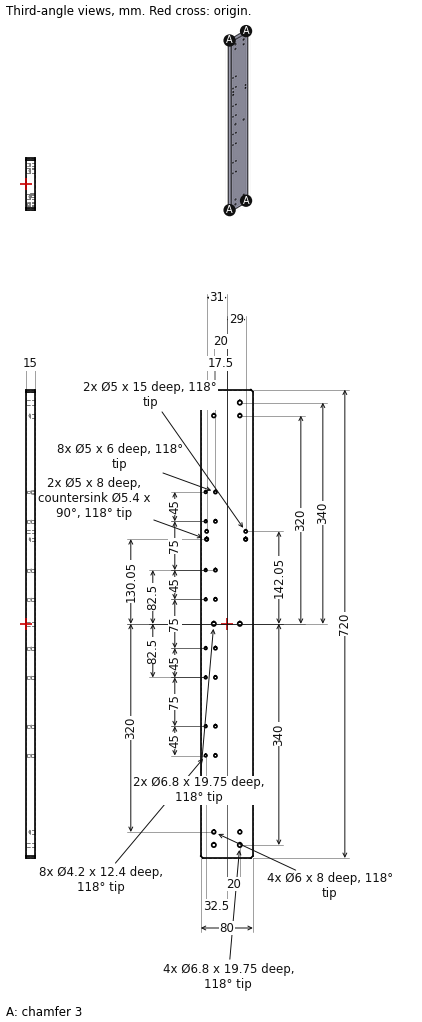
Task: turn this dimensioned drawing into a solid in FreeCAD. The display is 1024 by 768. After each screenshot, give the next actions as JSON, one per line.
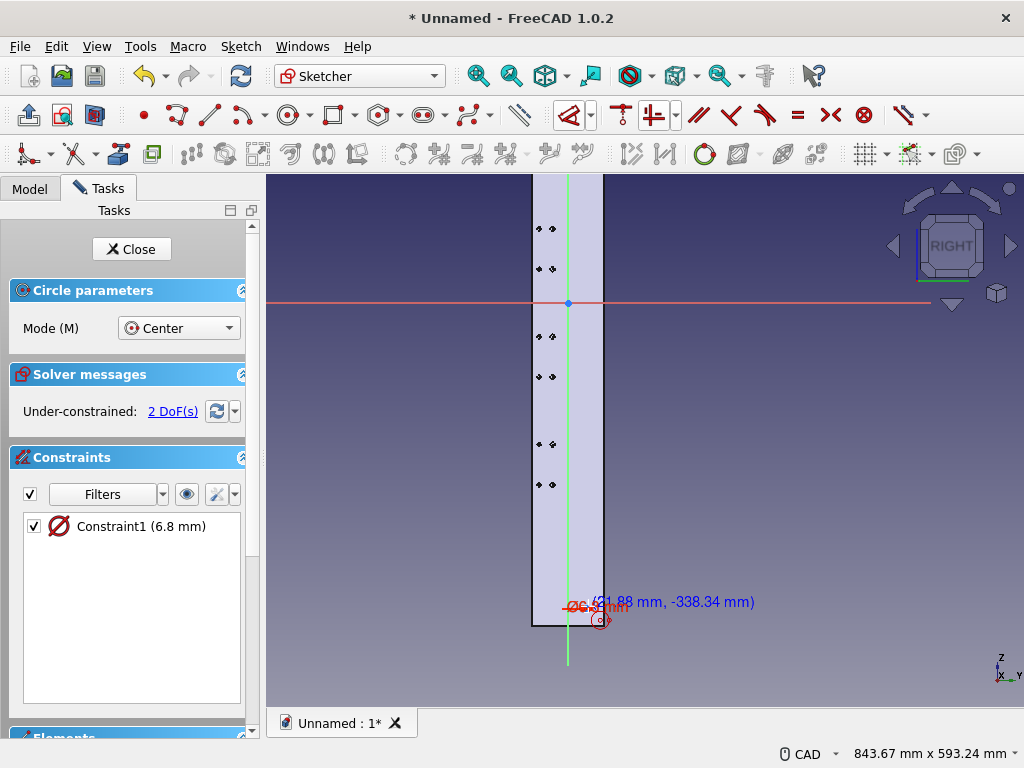
{"action": "scroll", "coordinate": [586, 608], "scroll_direction": "down", "scroll_amount": 3}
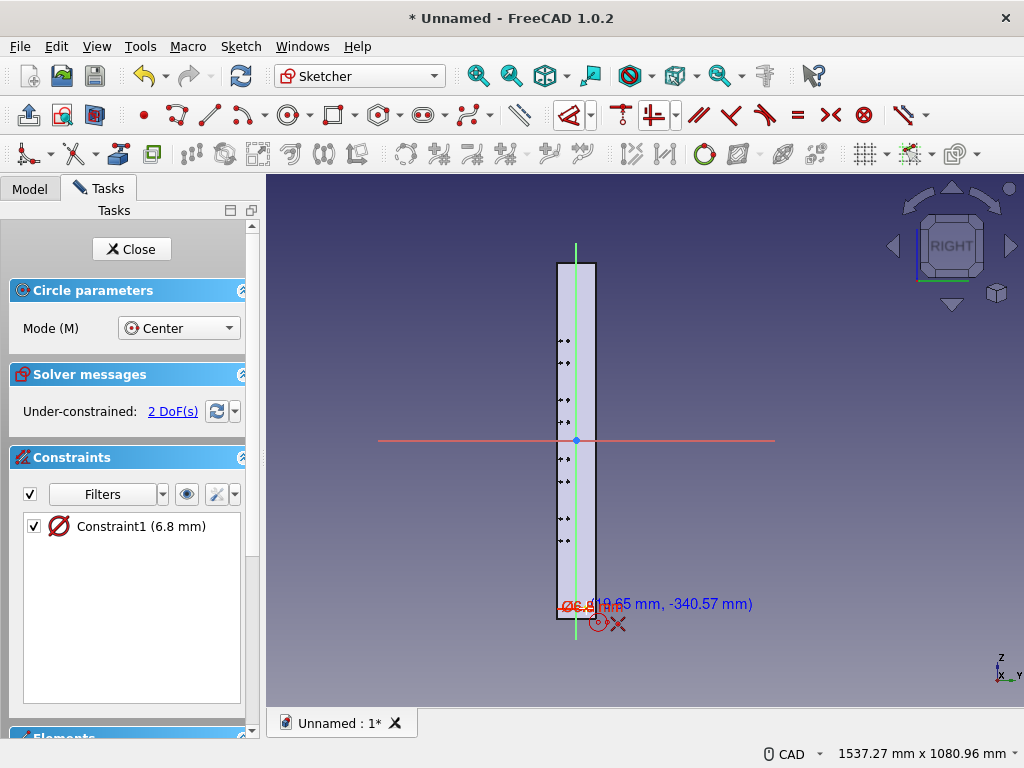
{"action": "scroll", "coordinate": [586, 273], "scroll_direction": "up", "scroll_amount": 14}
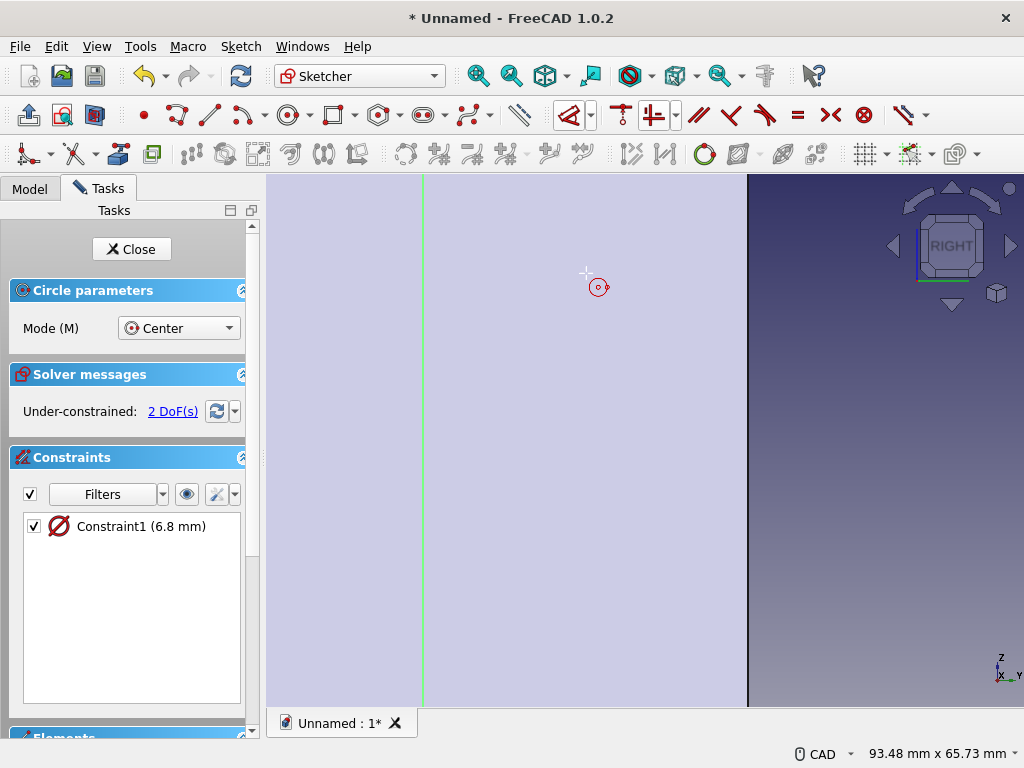
{"action": "scroll", "coordinate": [586, 273], "scroll_direction": "down", "scroll_amount": 14}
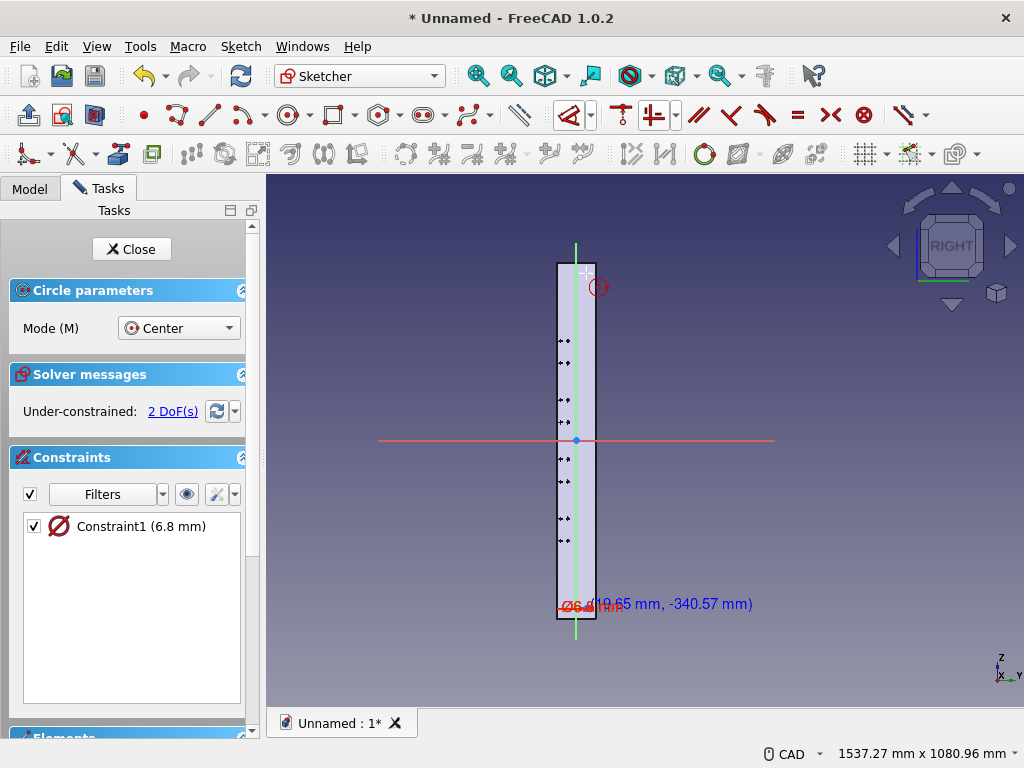
{"action": "scroll", "coordinate": [586, 273], "scroll_direction": "up", "scroll_amount": 3}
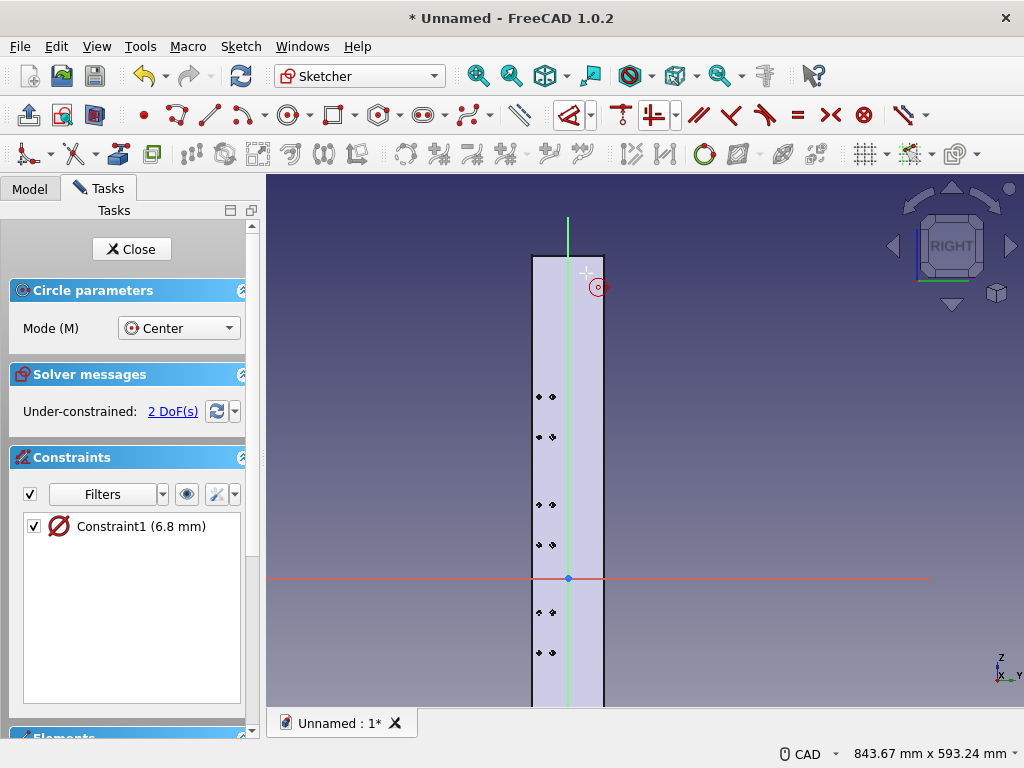
{"action": "left_click", "coordinate": [586, 273]}
{"action": "mouse_move", "coordinate": [588, 271]}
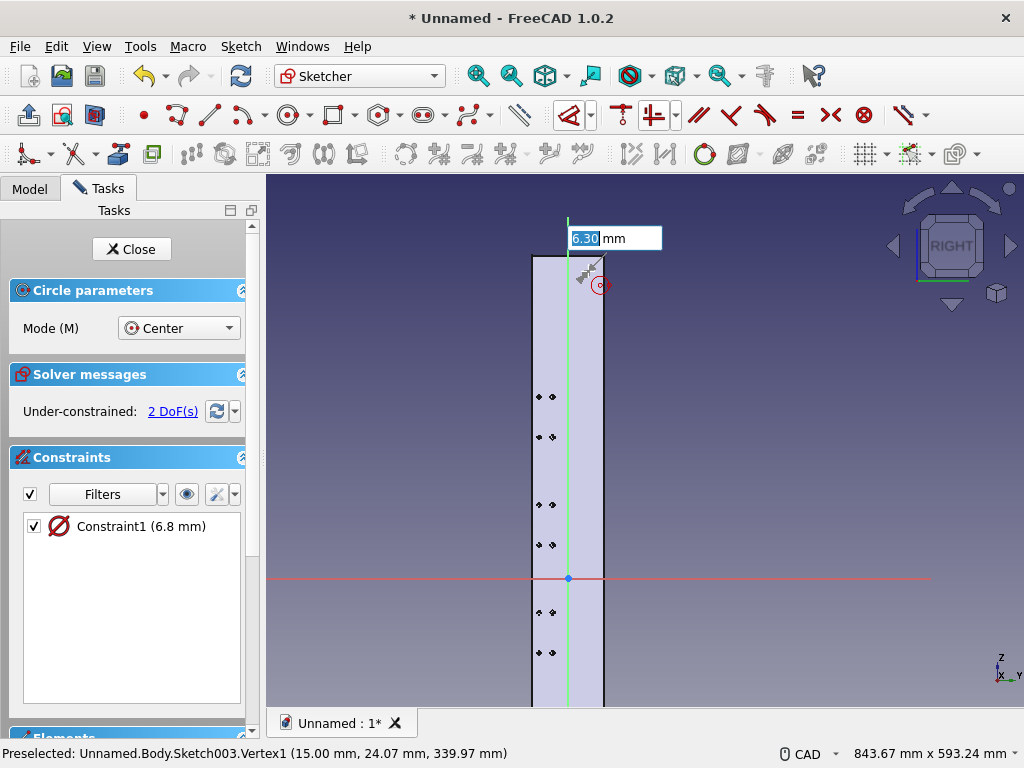
{"action": "type", "text": "6.8"}
{"action": "key", "text": "Return"}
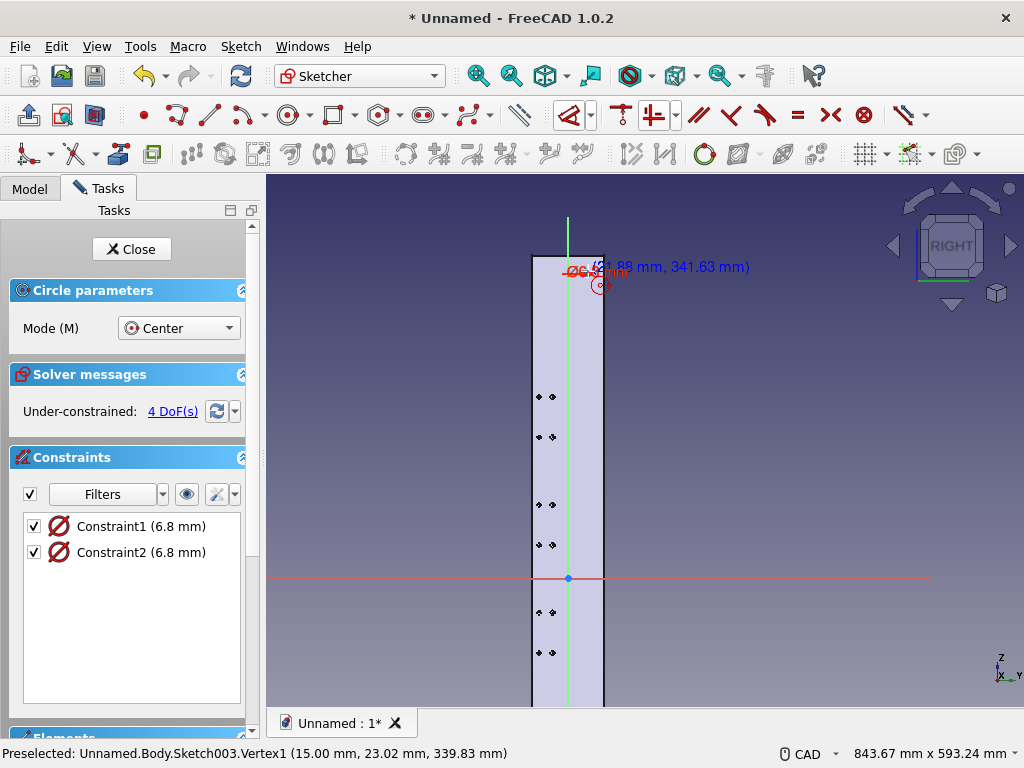
{"action": "scroll", "coordinate": [550, 273], "scroll_direction": "up", "scroll_amount": 11}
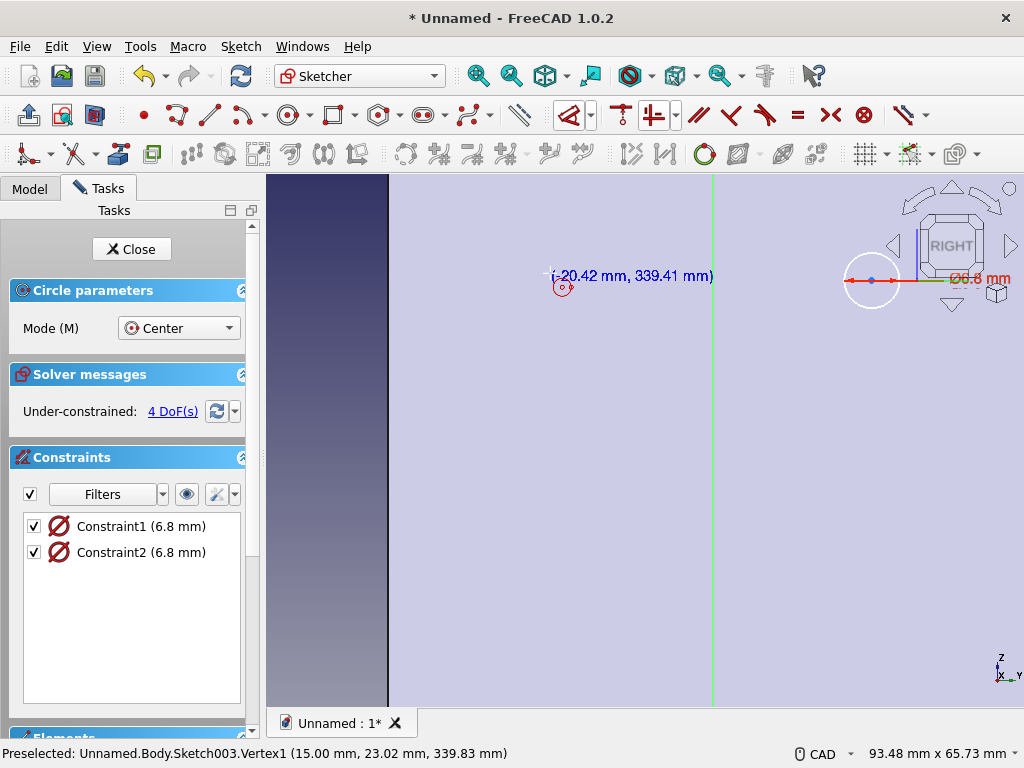
{"action": "scroll", "coordinate": [568, 273], "scroll_direction": "down", "scroll_amount": 14}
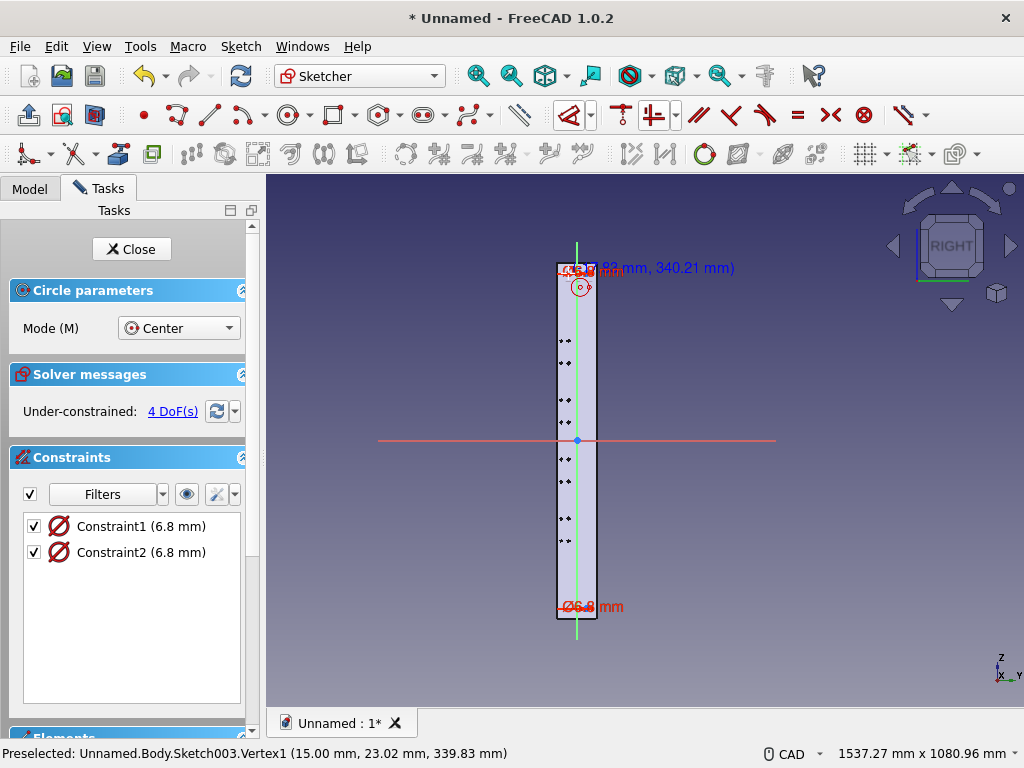
{"action": "scroll", "coordinate": [567, 273], "scroll_direction": "up", "scroll_amount": 3}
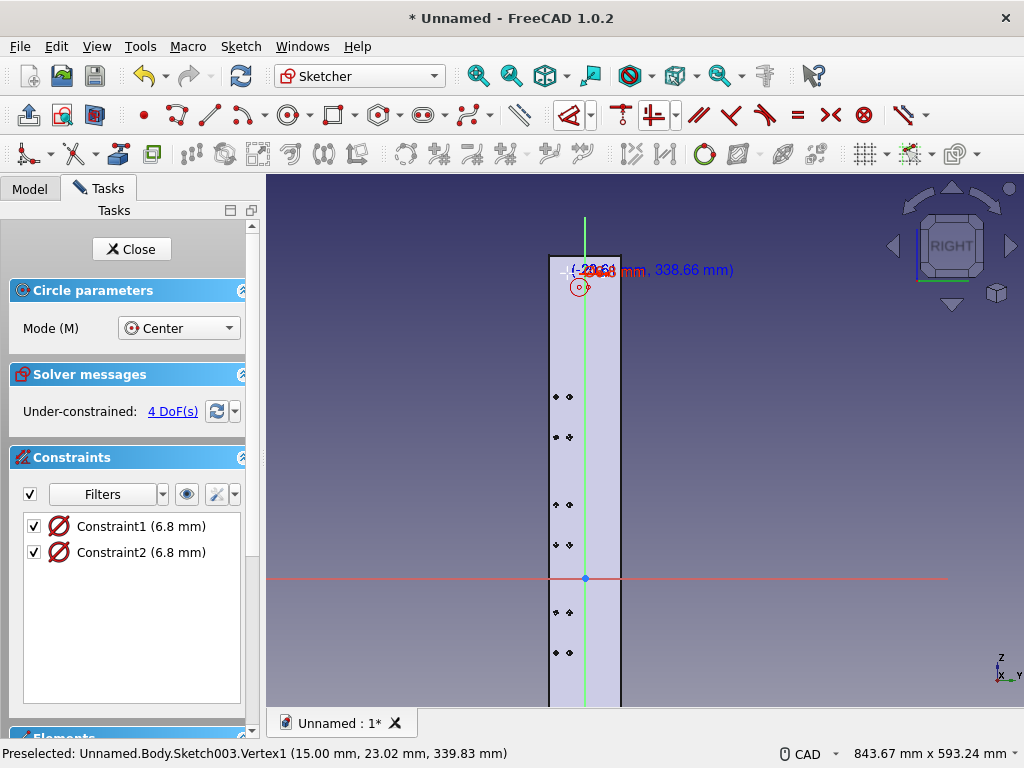
{"action": "left_click", "coordinate": [567, 273]}
{"action": "mouse_move", "coordinate": [569, 271]}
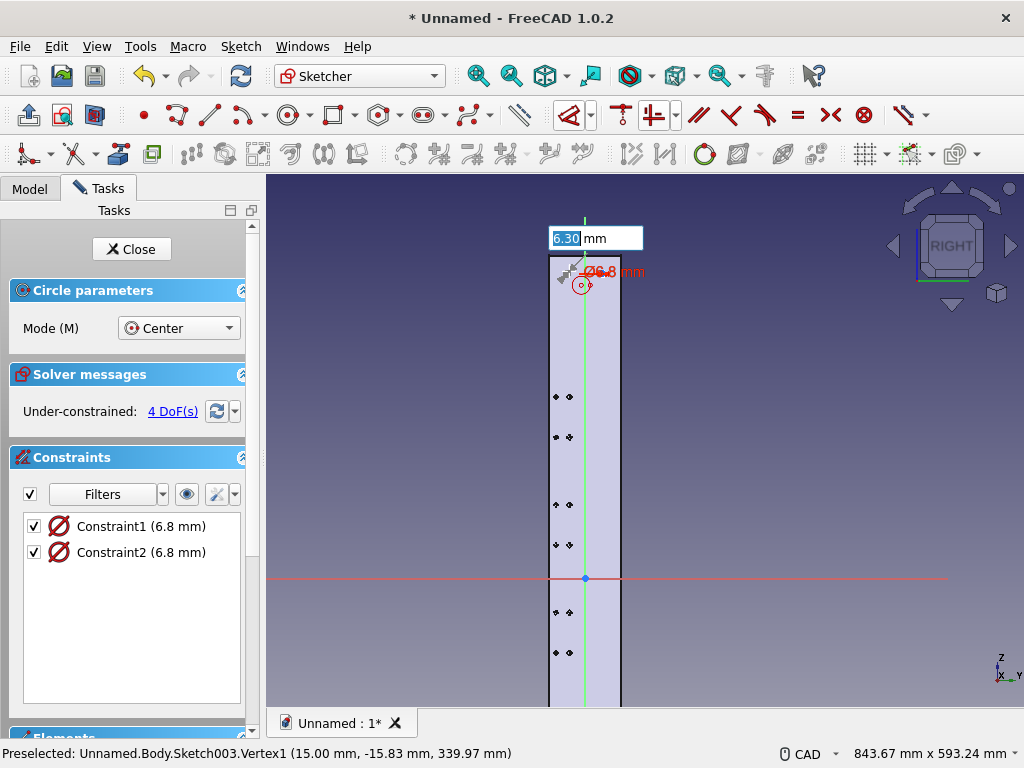
{"action": "type", "text": "6.8"}
{"action": "key", "text": "Return"}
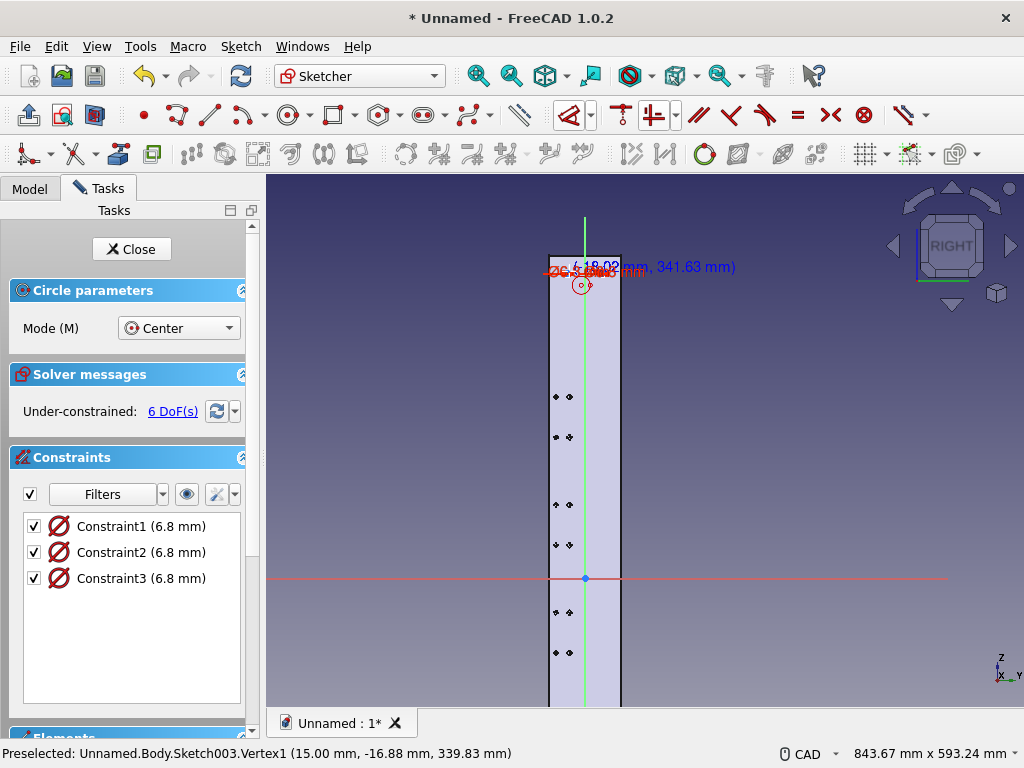
{"action": "scroll", "coordinate": [566, 272], "scroll_direction": "down", "scroll_amount": 3}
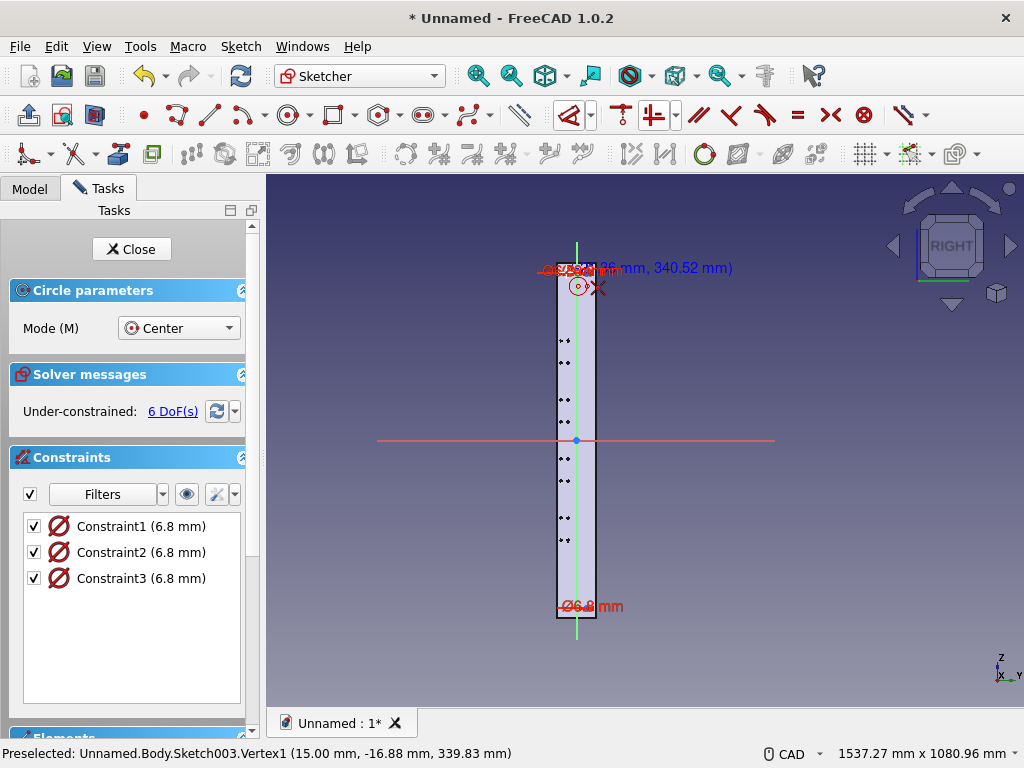
{"action": "scroll", "coordinate": [567, 608], "scroll_direction": "up", "scroll_amount": 14}